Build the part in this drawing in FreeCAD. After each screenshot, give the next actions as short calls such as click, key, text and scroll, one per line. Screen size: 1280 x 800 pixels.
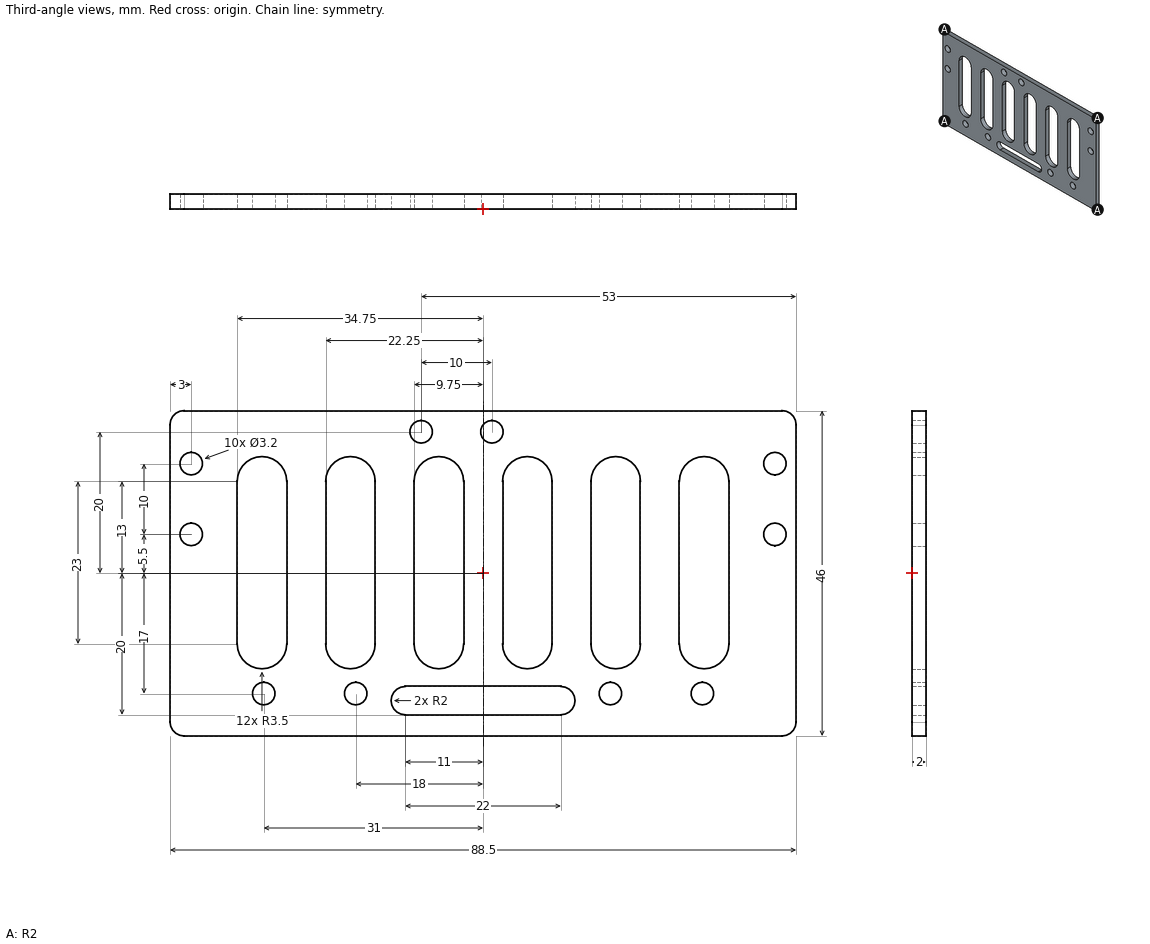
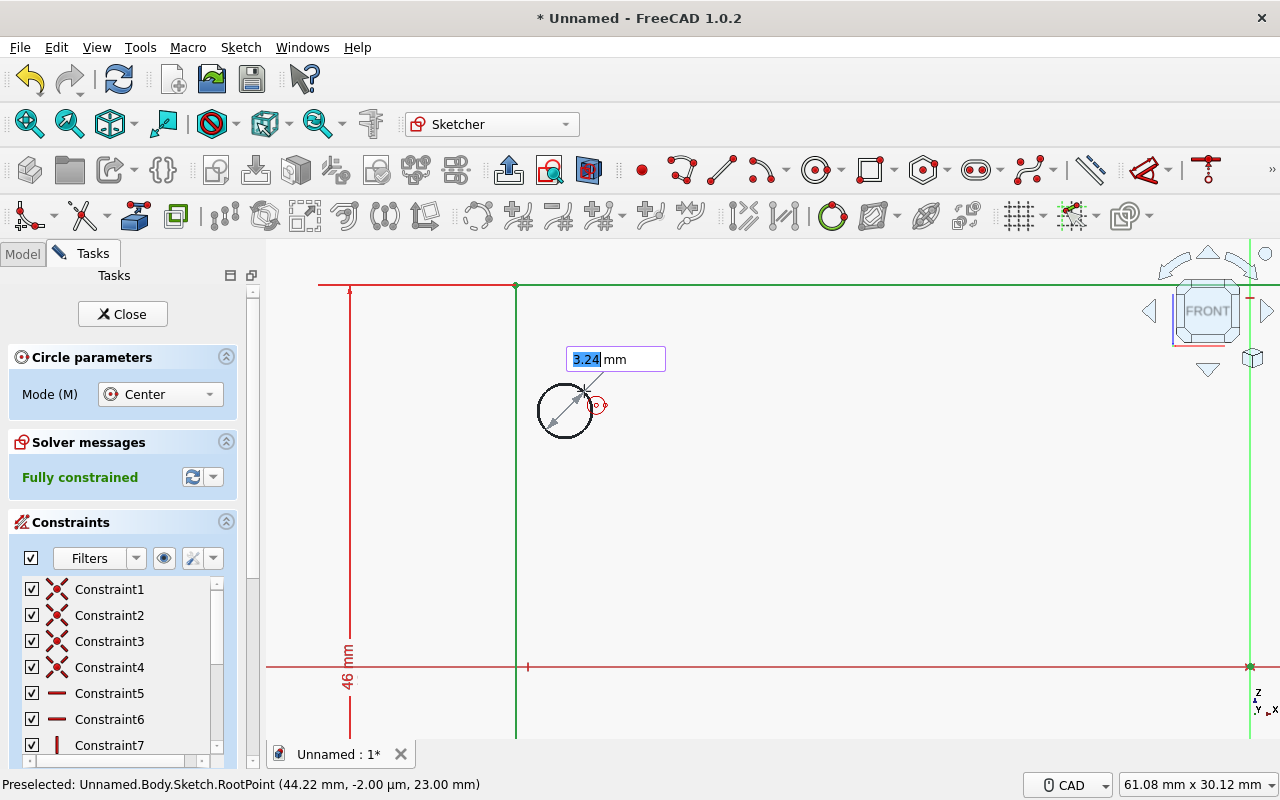
text(3.2)
key(Return)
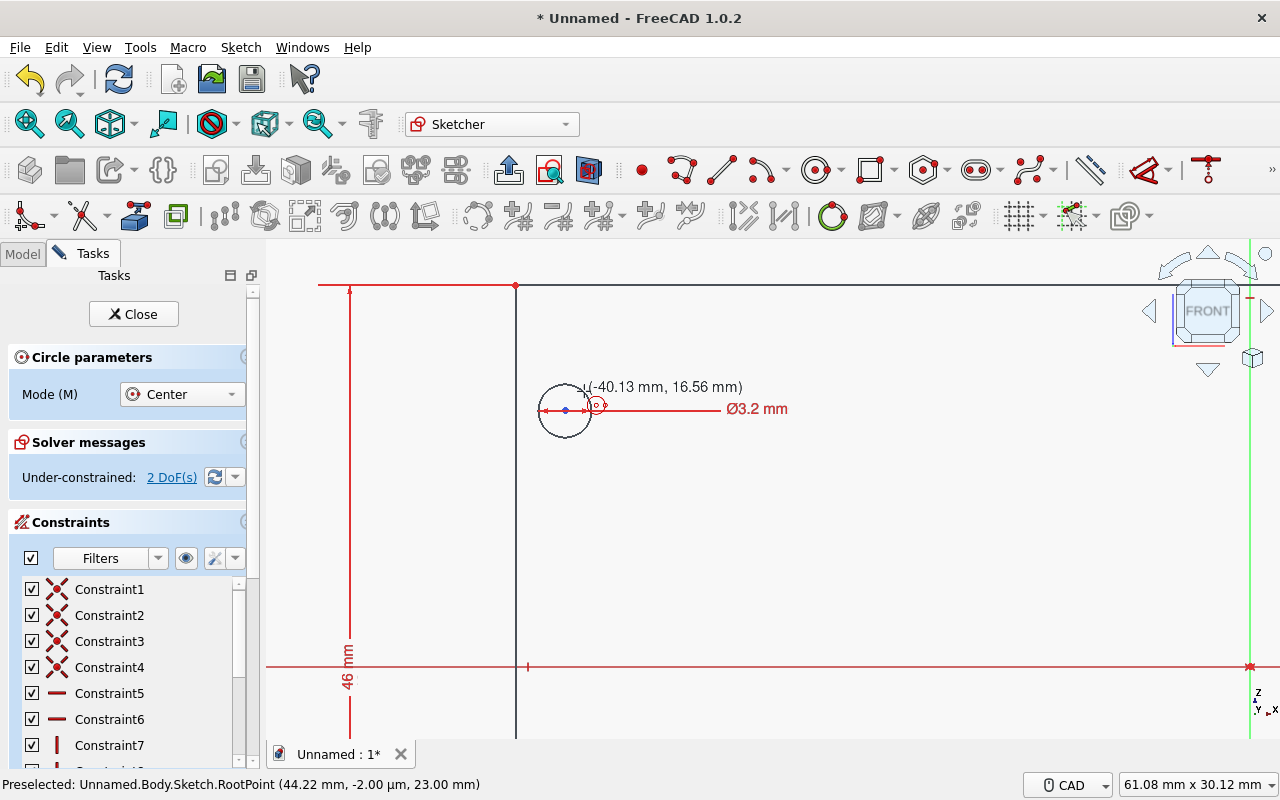
click(1105, 335)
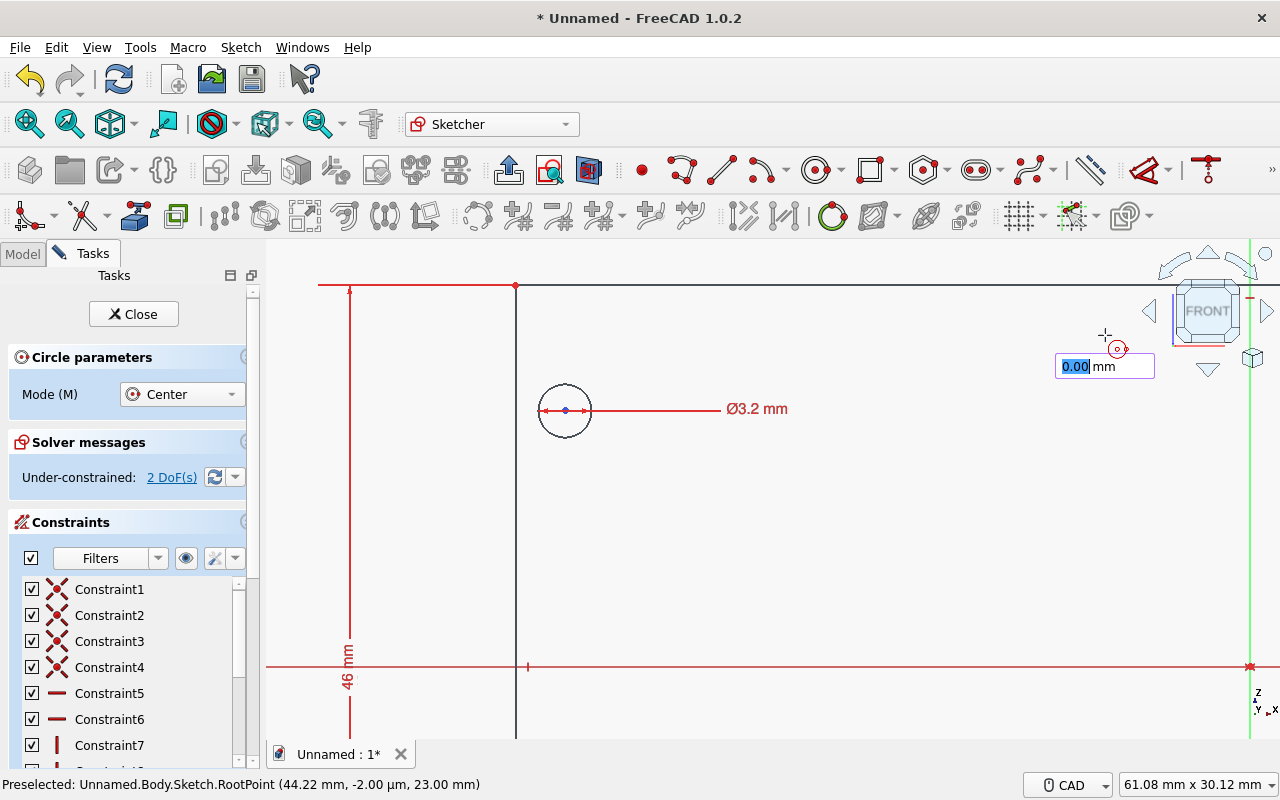
scroll(387, 385, down, 5)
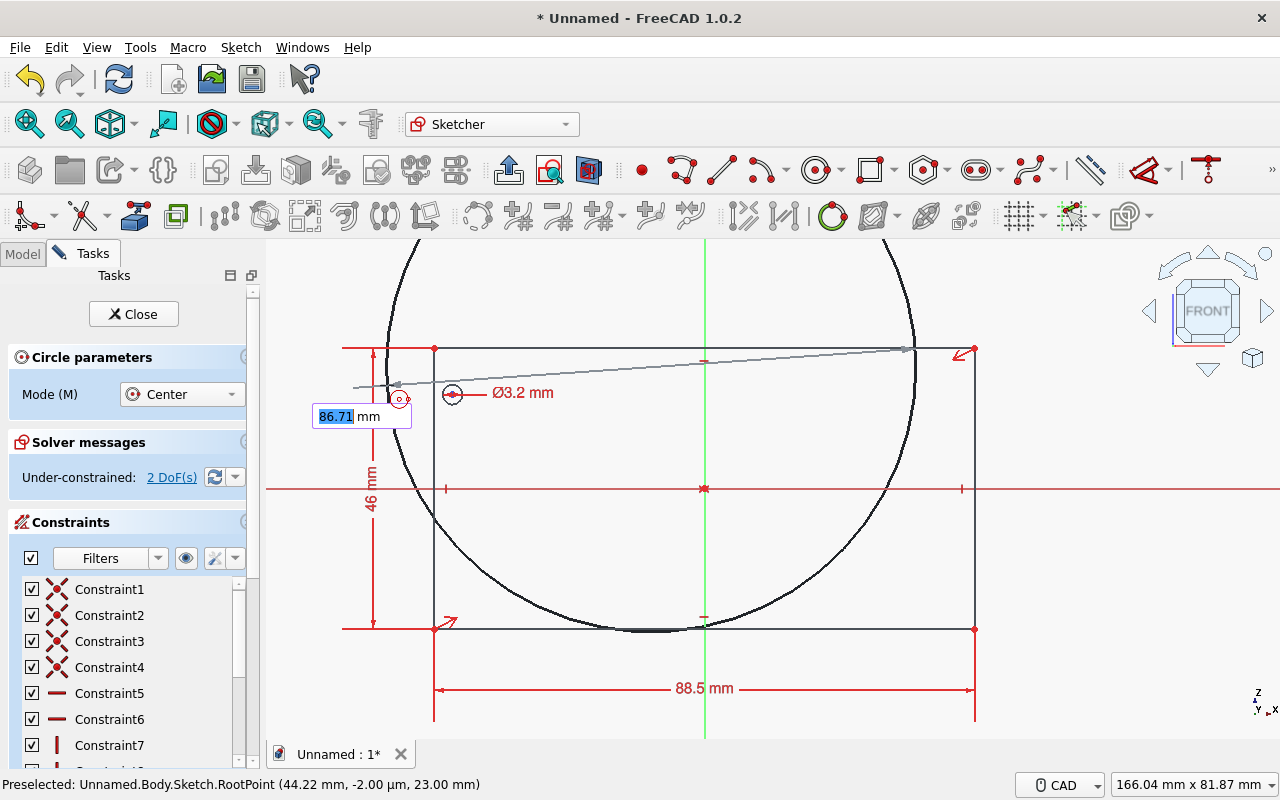
scroll(658, 360, up, 2)
move(658, 360)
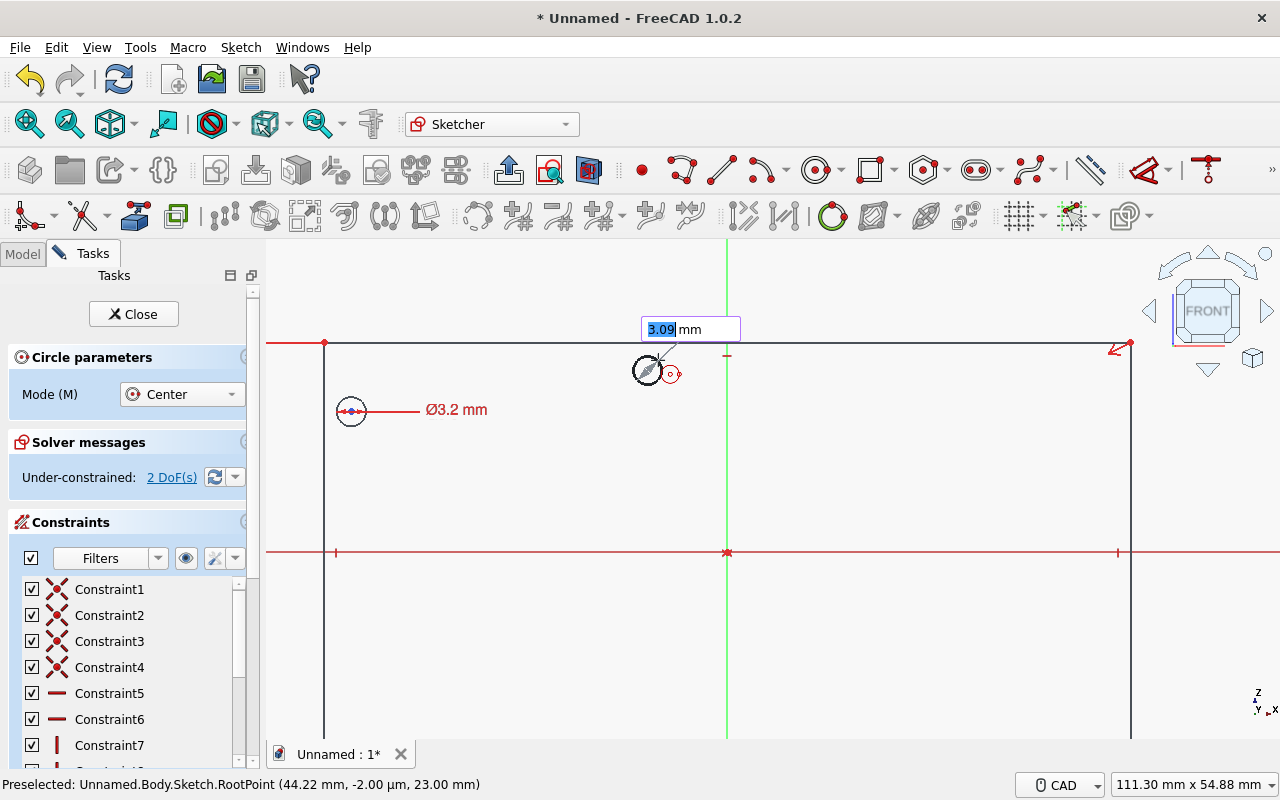
text(3.2)
key(Return)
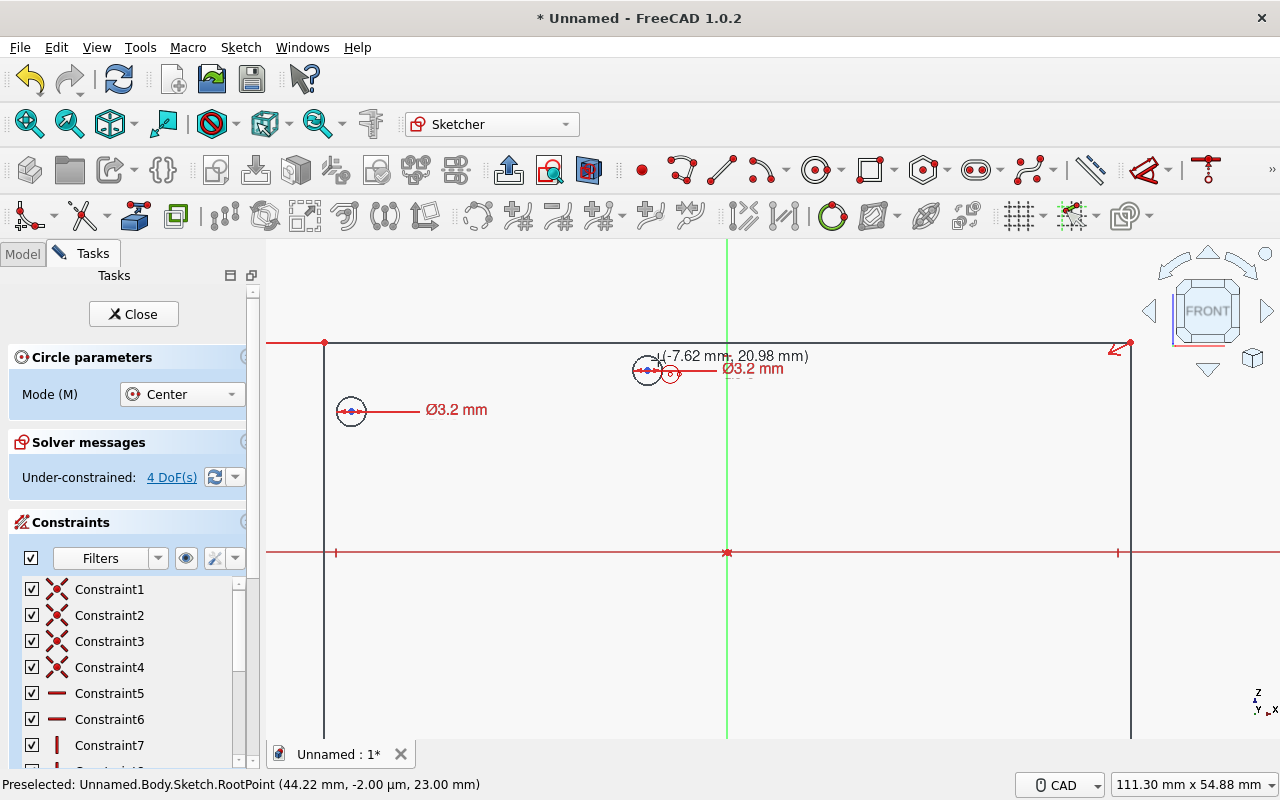
scroll(352, 502, up, 3)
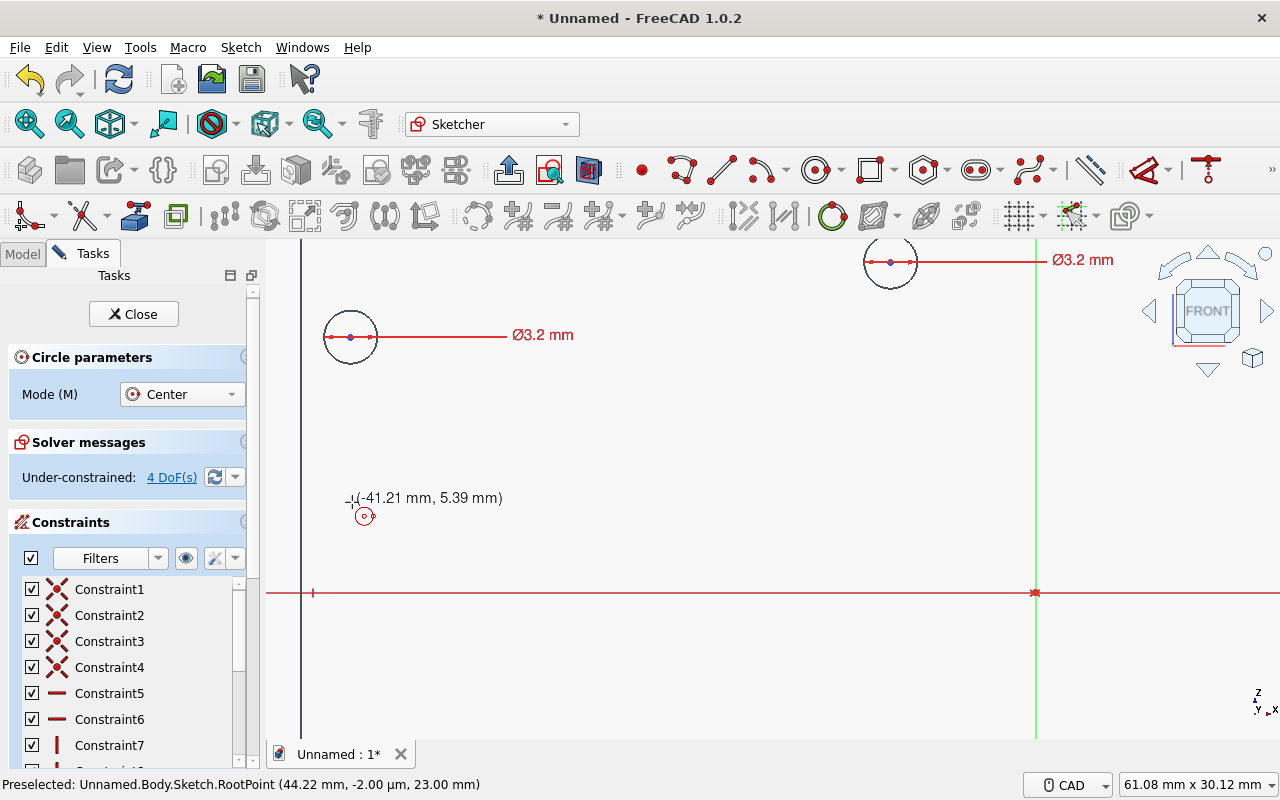
click(351, 502)
move(370, 483)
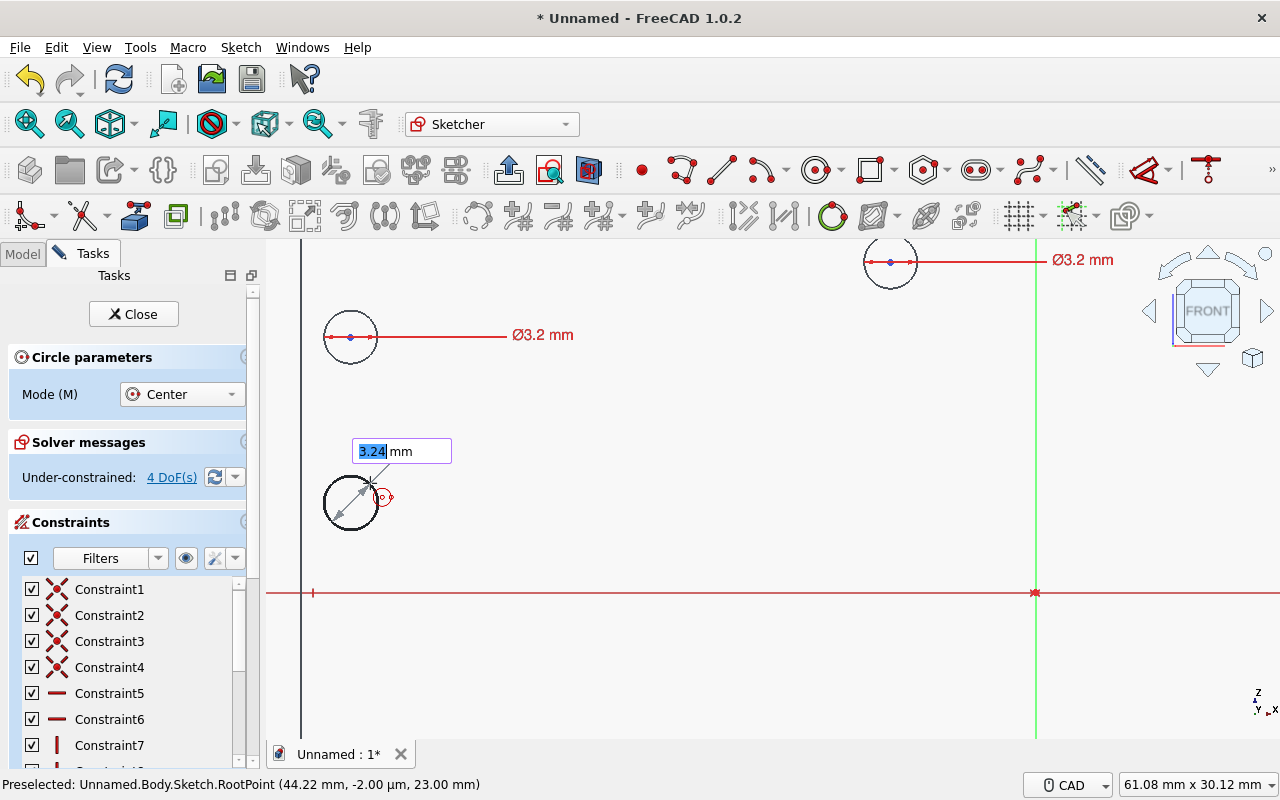
text(3.2)
key(Return)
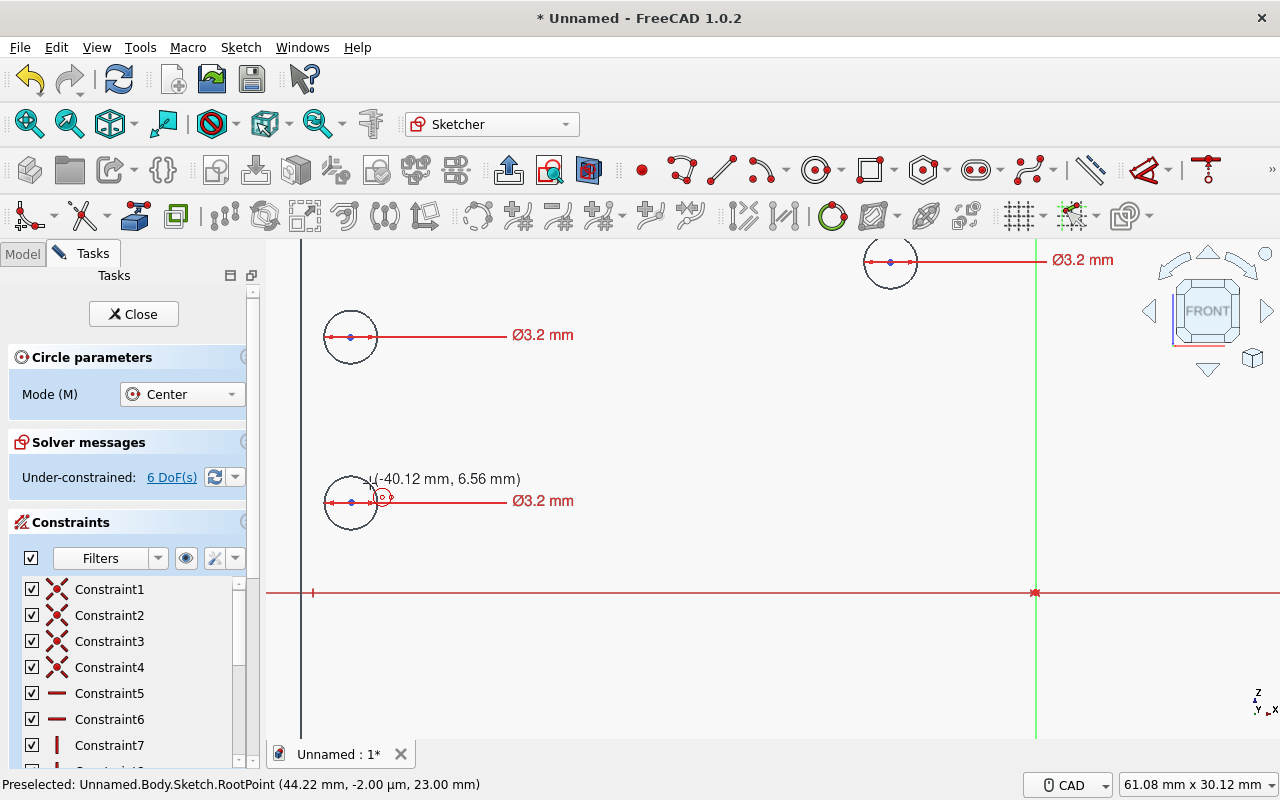
scroll(512, 429, down, 5)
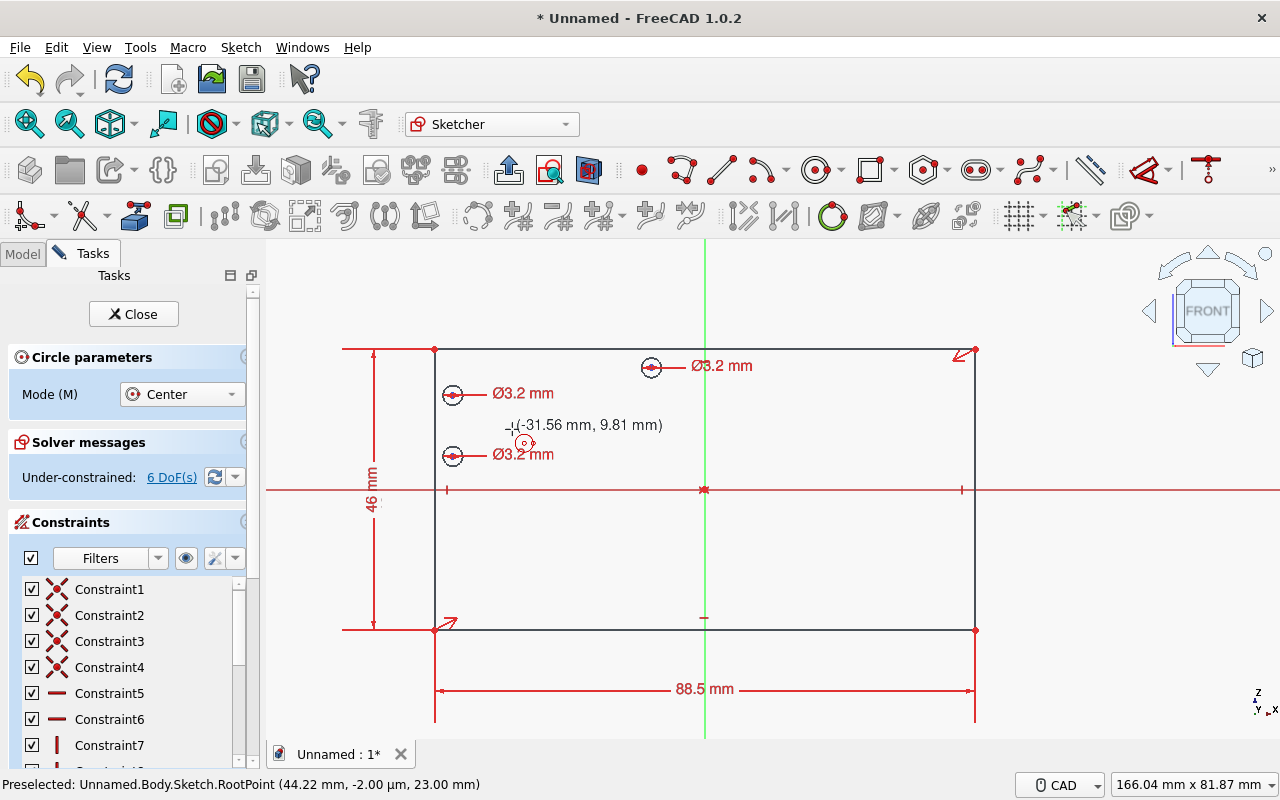
scroll(713, 367, up, 5)